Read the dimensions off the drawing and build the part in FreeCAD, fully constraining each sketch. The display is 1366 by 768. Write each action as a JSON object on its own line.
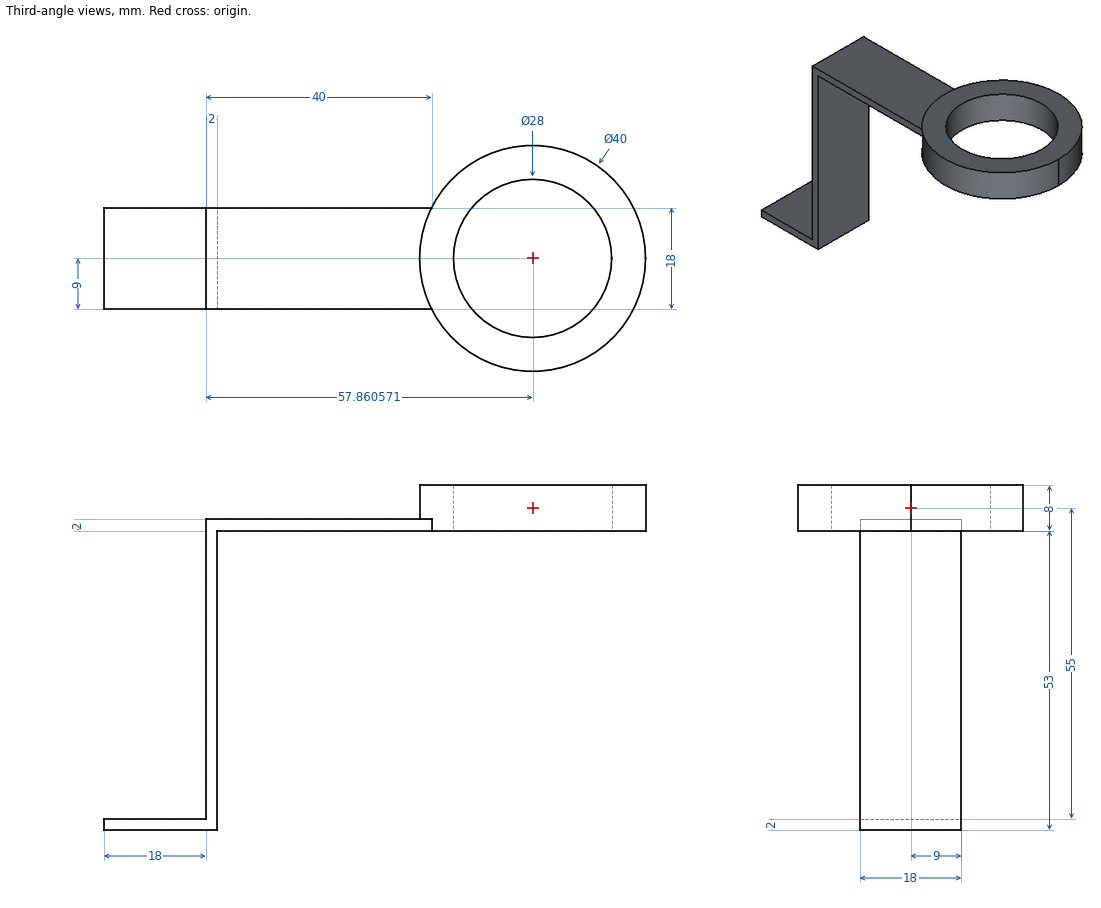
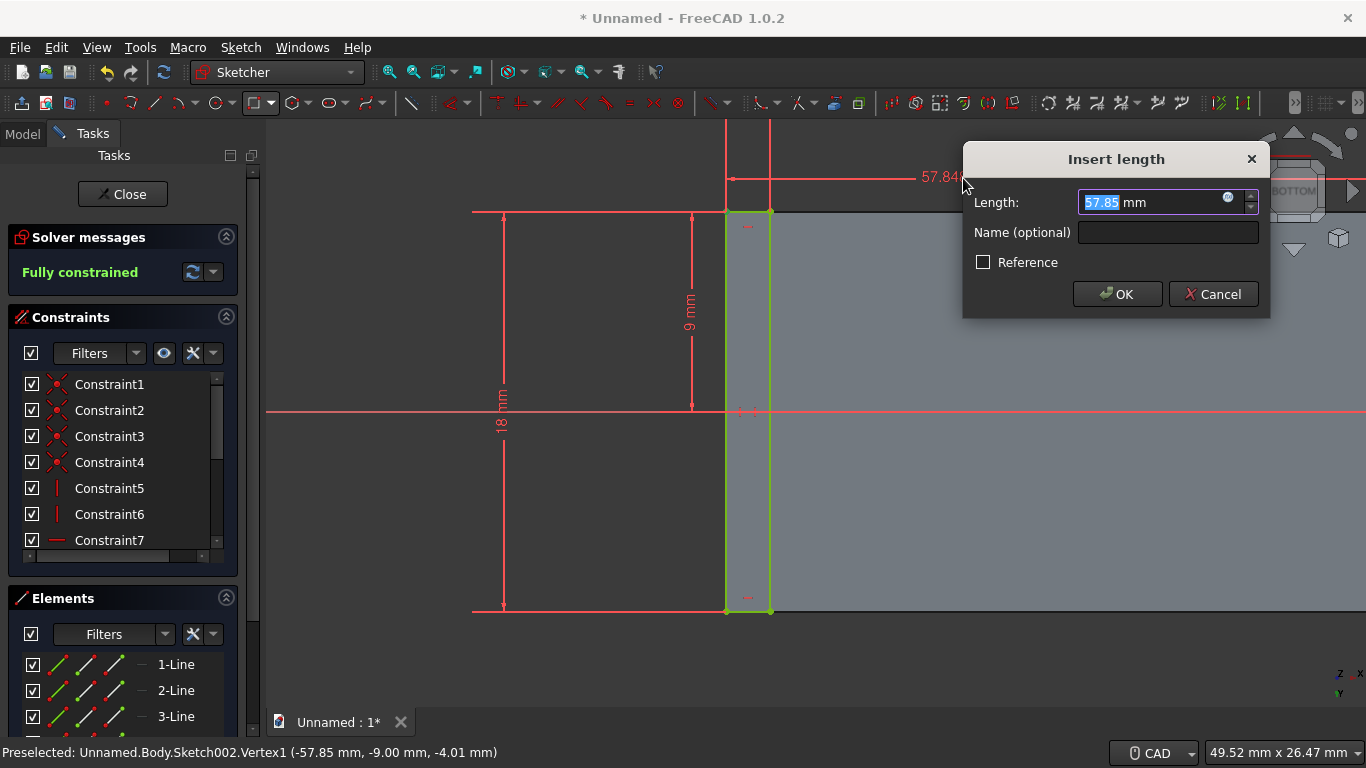
{"action": "type", "text": "57.860571"}
{"action": "key", "text": "Return"}
{"action": "key", "text": "Escape"}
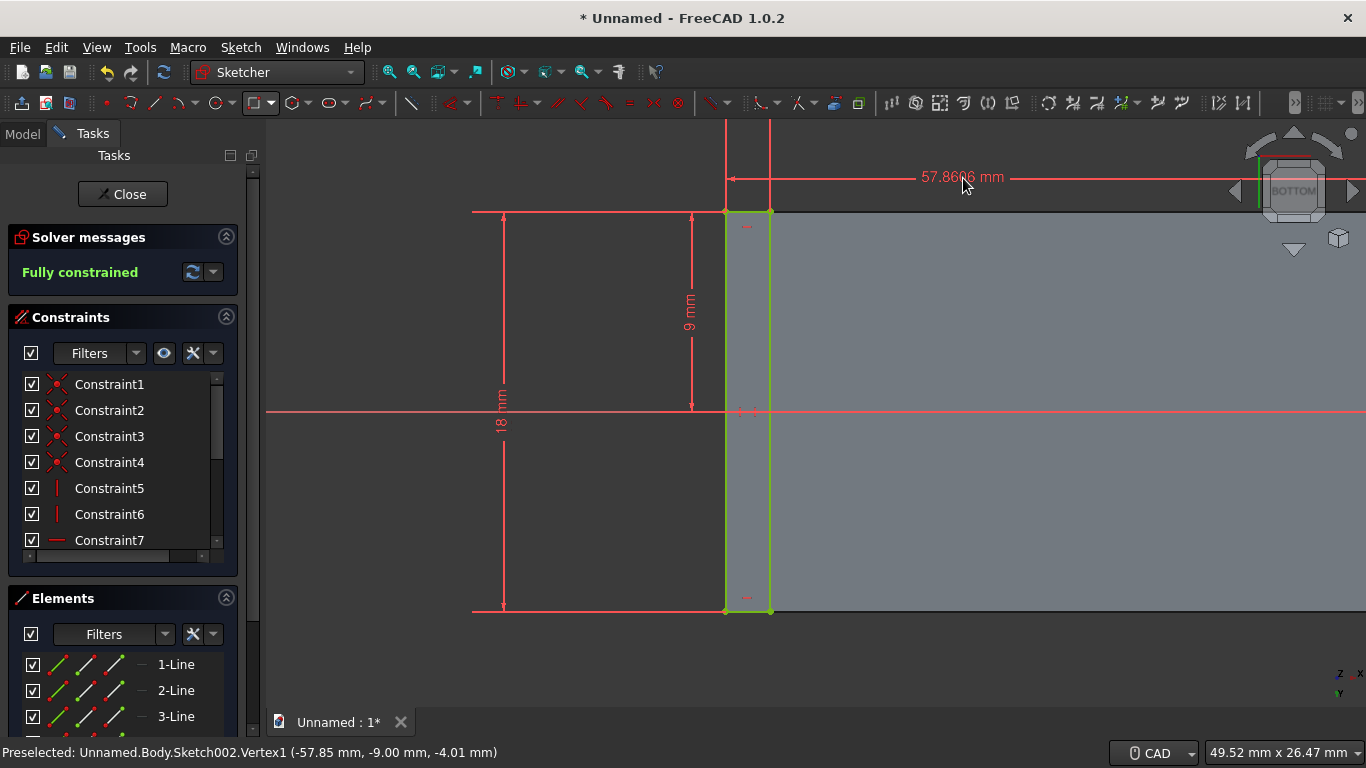
{"action": "left_click", "coordinate": [123, 194]}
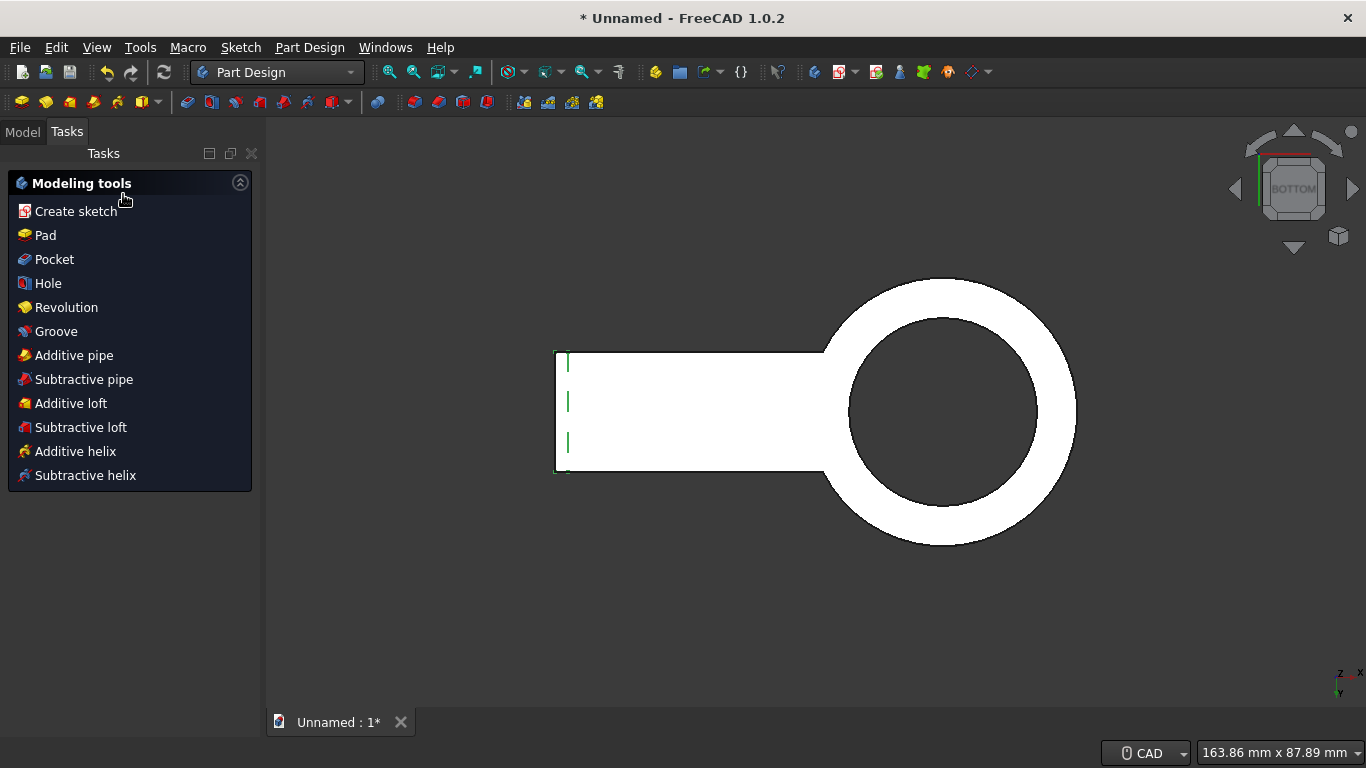
{"action": "left_click", "coordinate": [22, 102]}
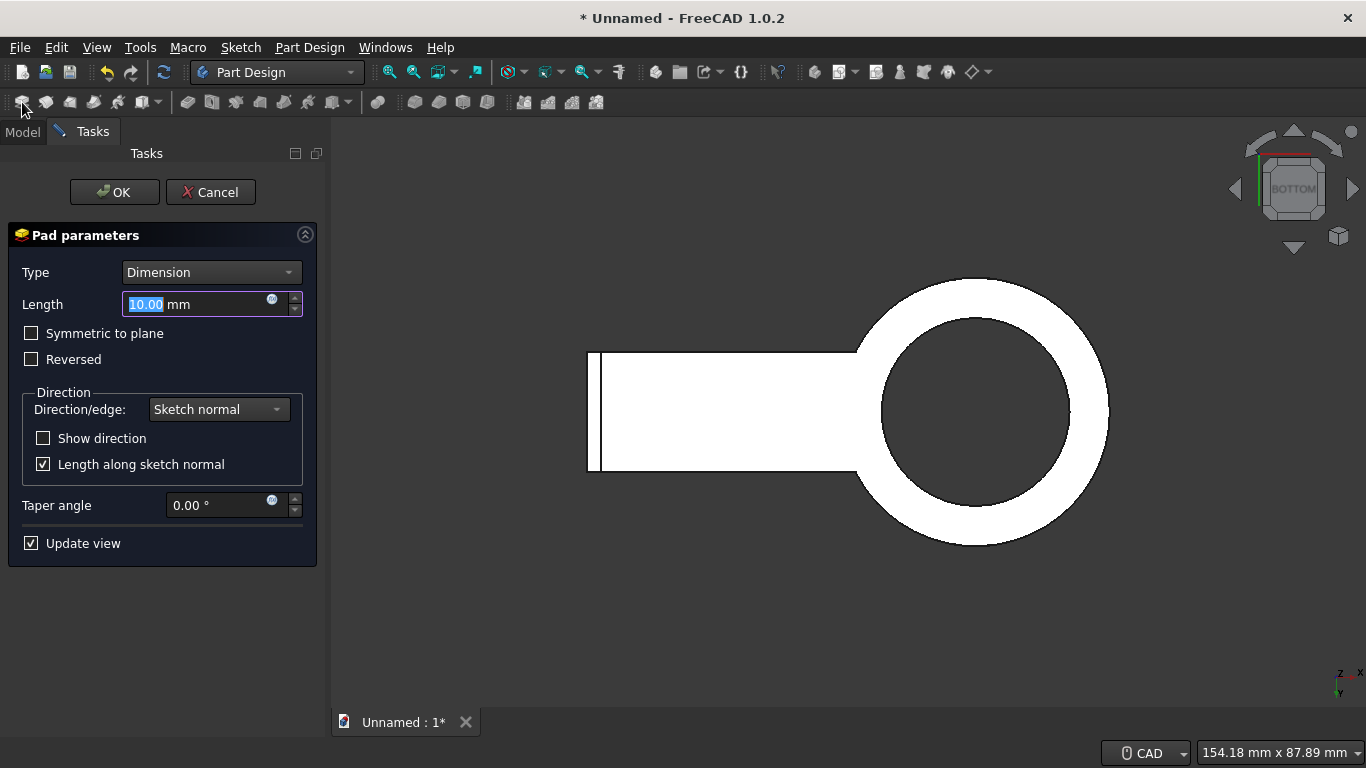
{"action": "type", "text": "53"}
{"action": "key", "text": "Tab"}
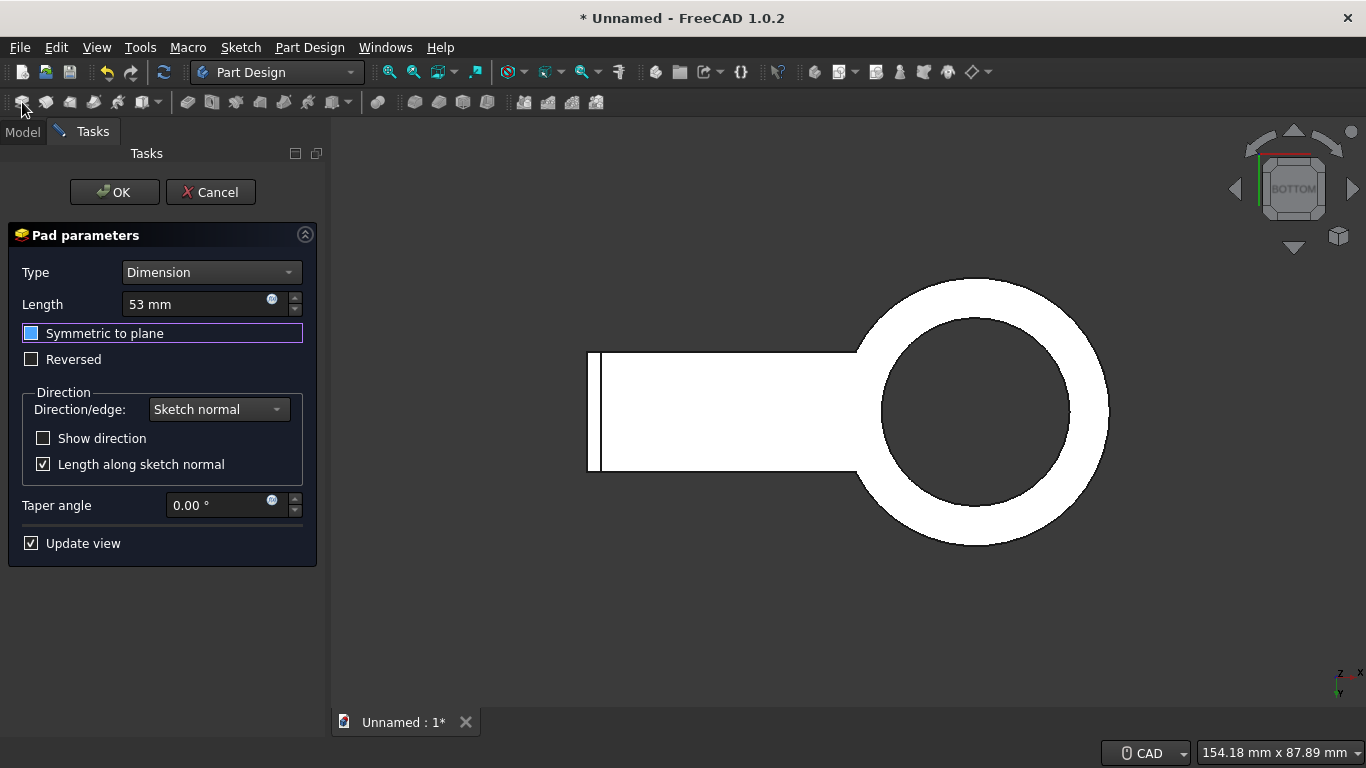
{"action": "left_click", "coordinate": [115, 192]}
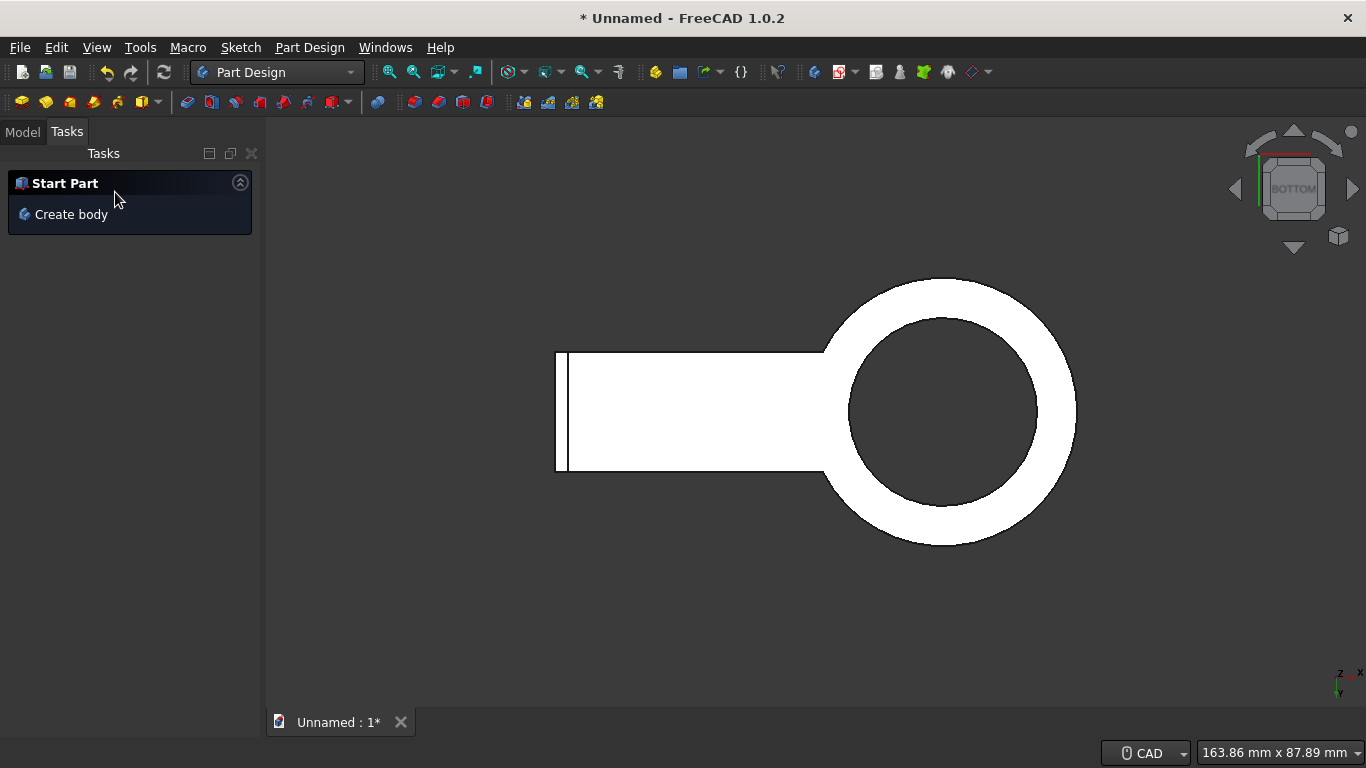
{"action": "key", "text": "6"}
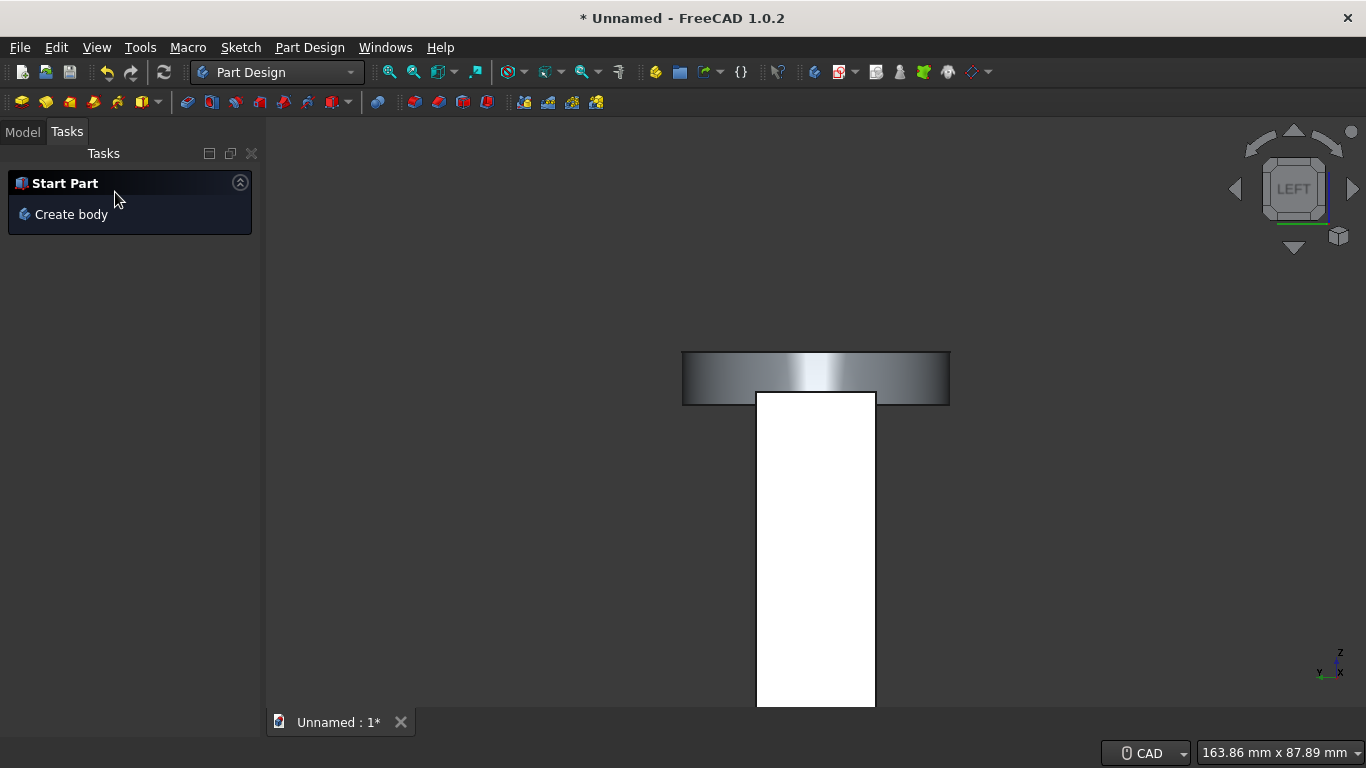
{"action": "left_click", "coordinate": [390, 72]}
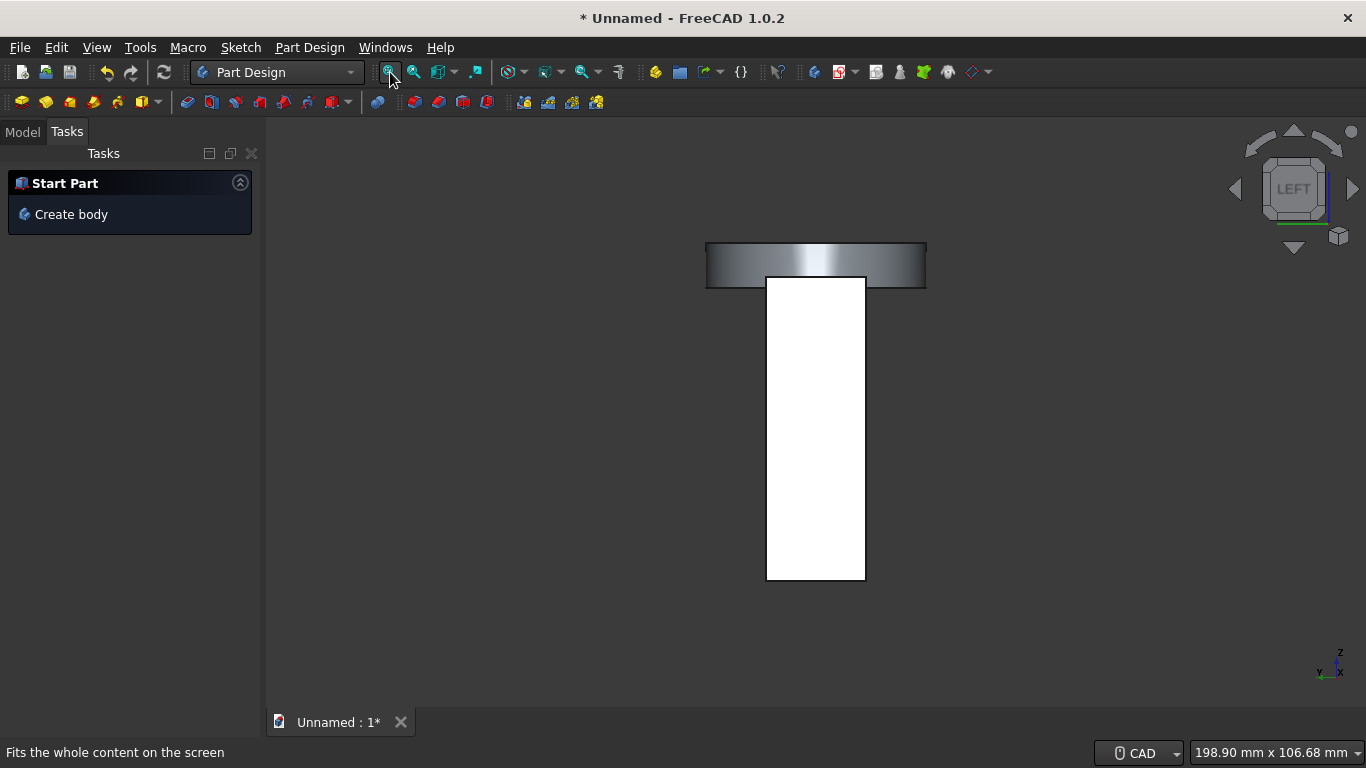
{"action": "left_click", "coordinate": [816, 341]}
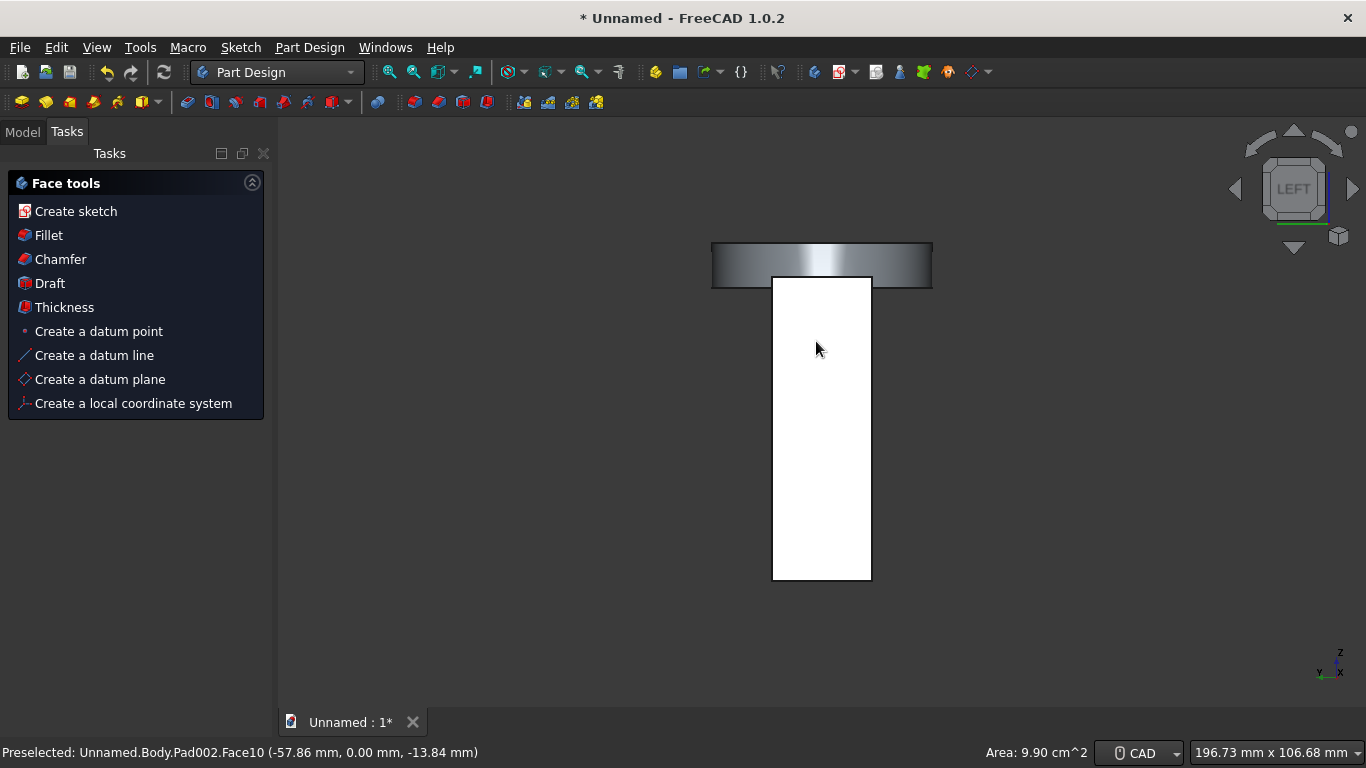
{"action": "left_click", "coordinate": [840, 72]}